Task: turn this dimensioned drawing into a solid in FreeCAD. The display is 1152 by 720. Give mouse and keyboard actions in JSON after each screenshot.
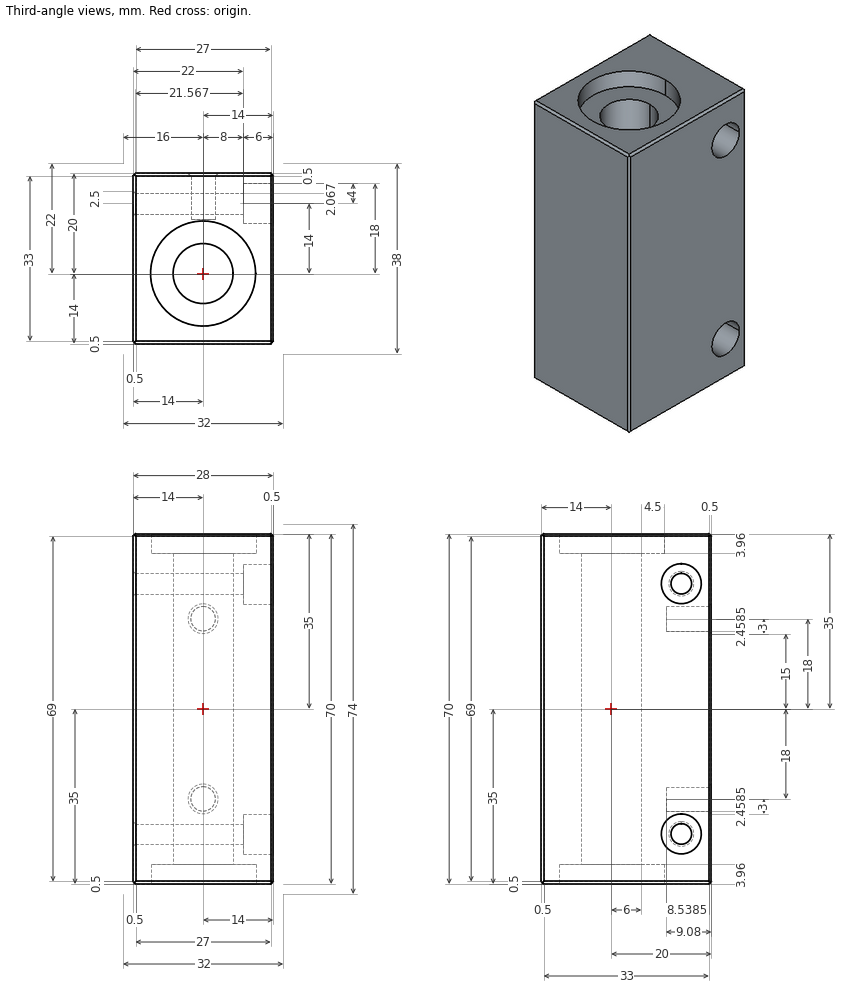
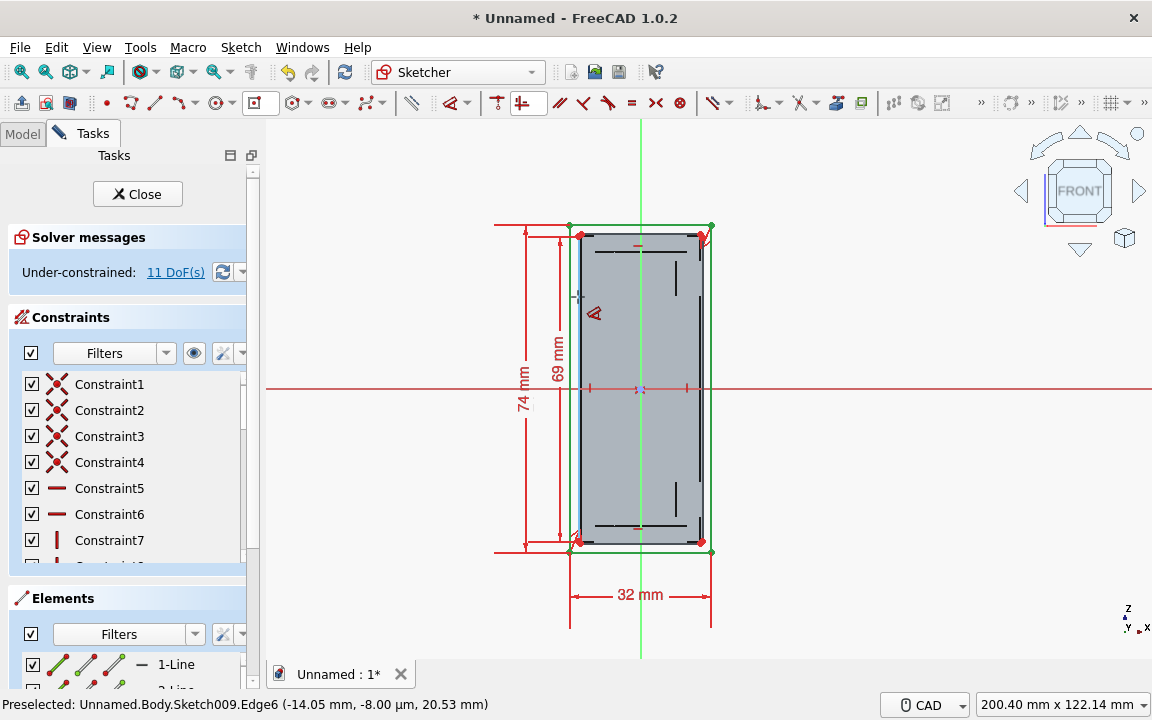
{"action": "scroll", "coordinate": [617, 544], "scroll_direction": "up", "scroll_amount": 3}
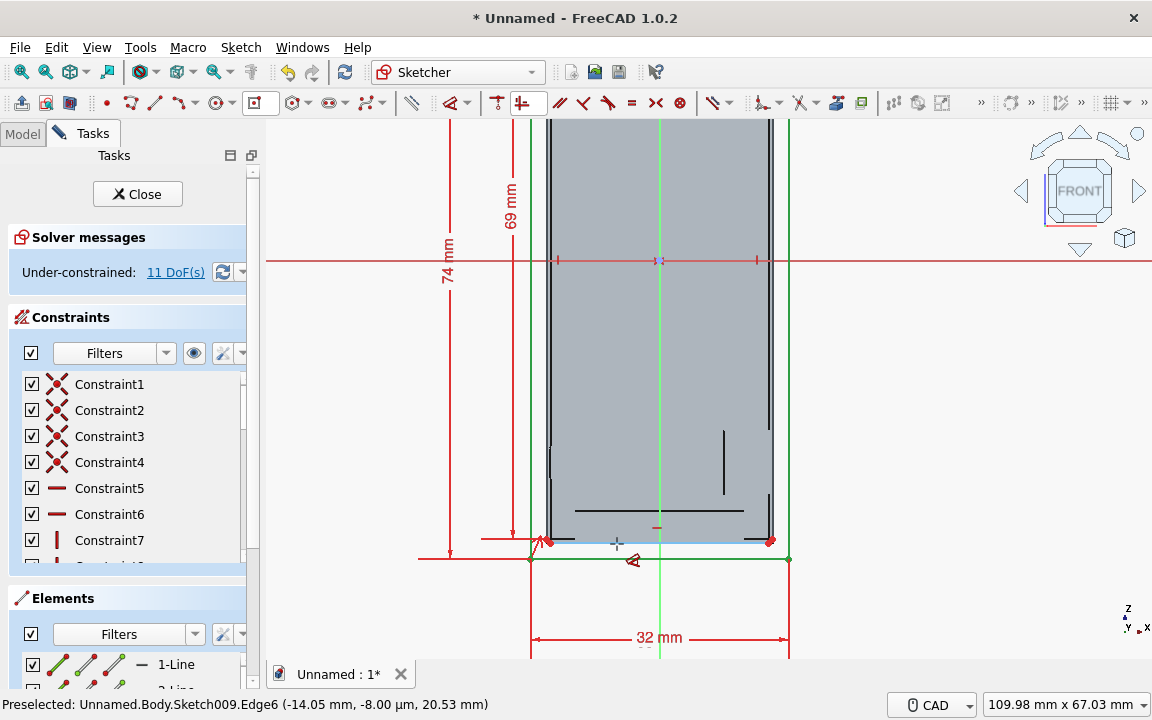
{"action": "left_click", "coordinate": [616, 543]}
{"action": "left_click", "coordinate": [610, 577]}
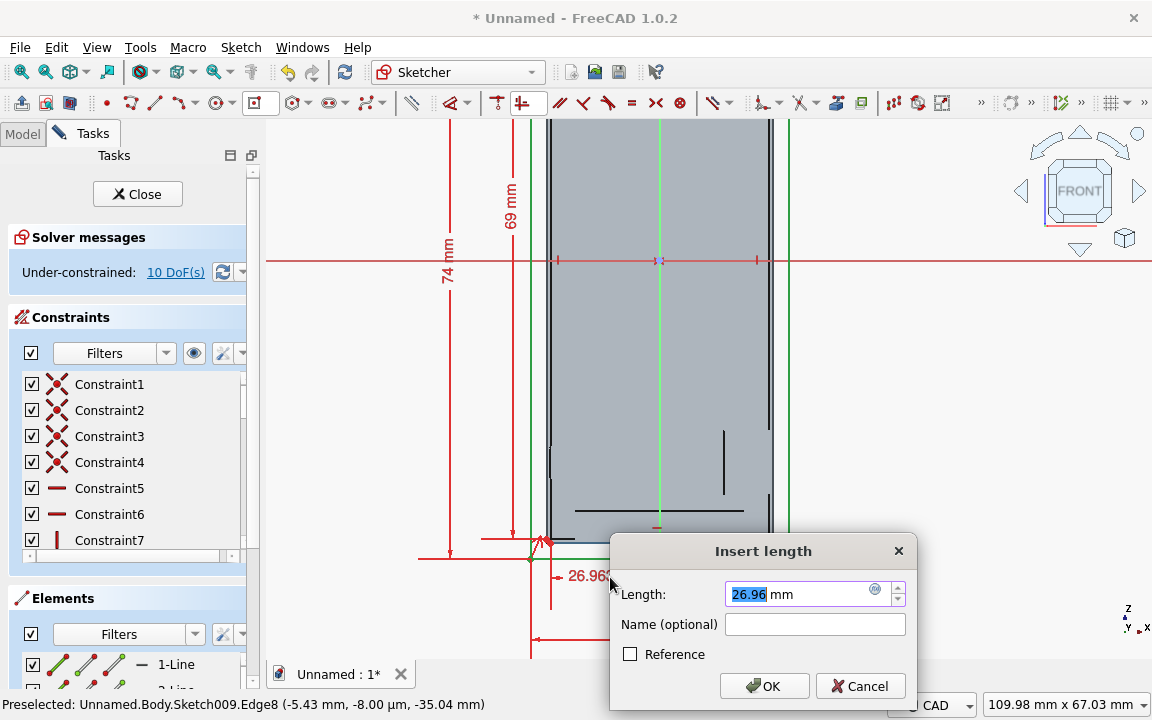
{"action": "type", "text": "27"}
{"action": "key", "text": "Return"}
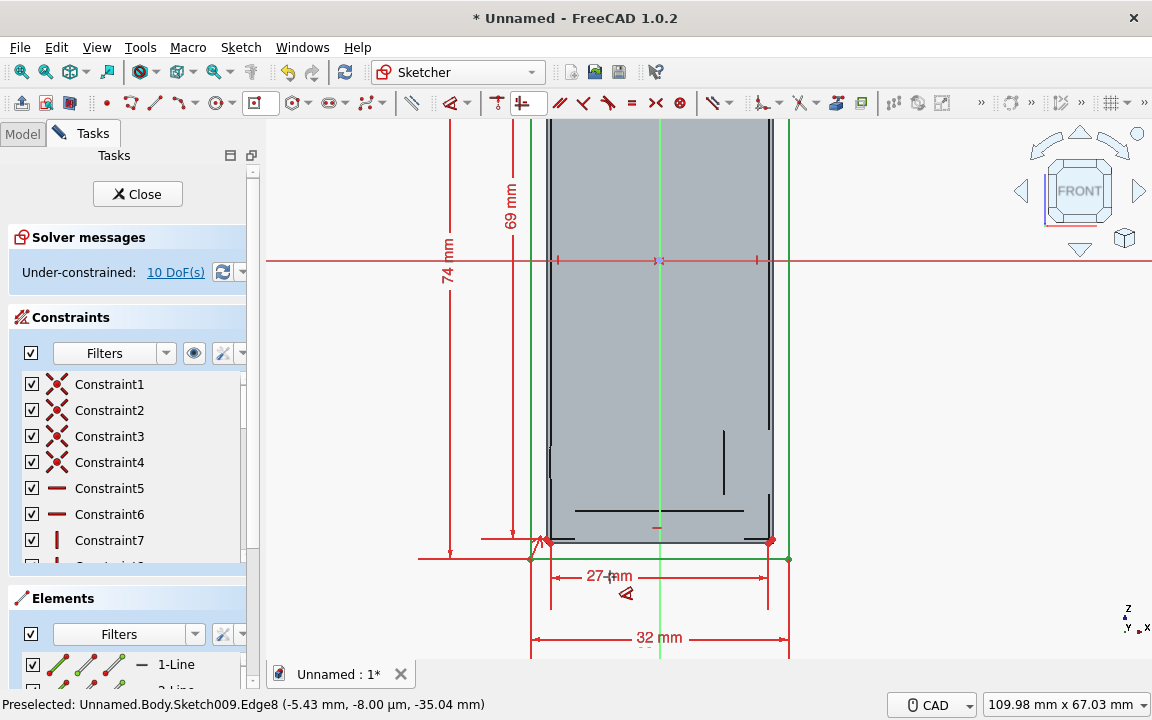
{"action": "left_click", "coordinate": [773, 373]}
{"action": "left_click", "coordinate": [807, 343]}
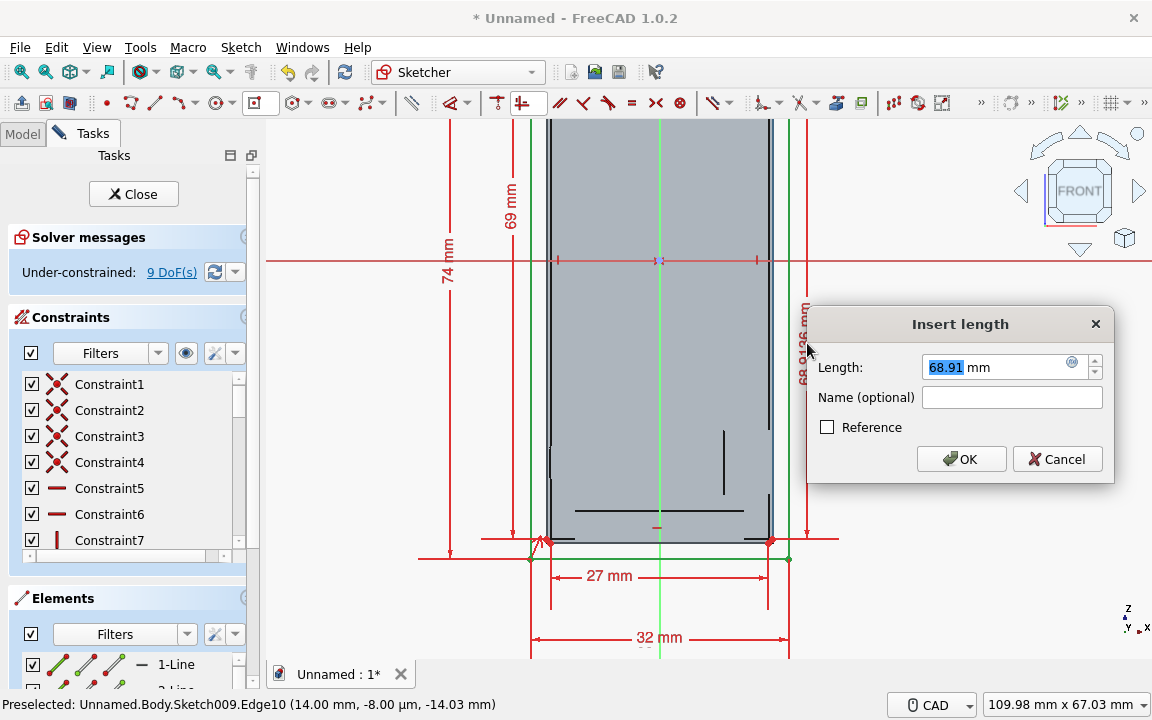
{"action": "type", "text": "69"}
{"action": "key", "text": "Return"}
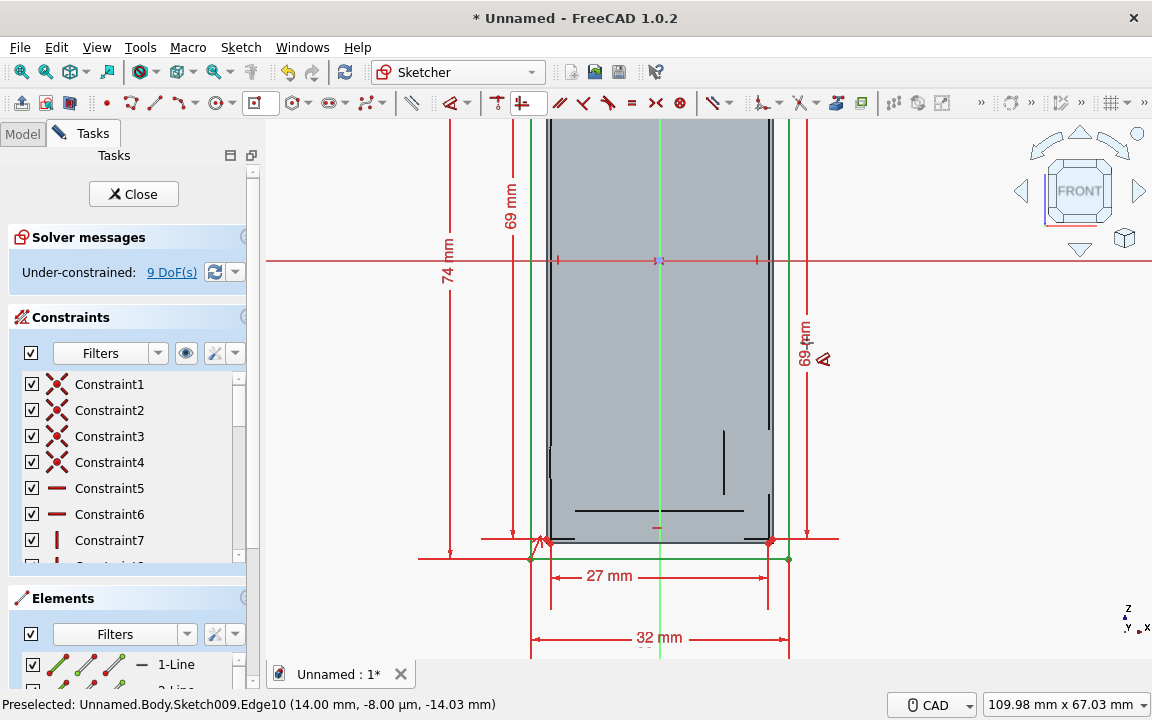
{"action": "scroll", "coordinate": [617, 545], "scroll_direction": "down", "scroll_amount": 3}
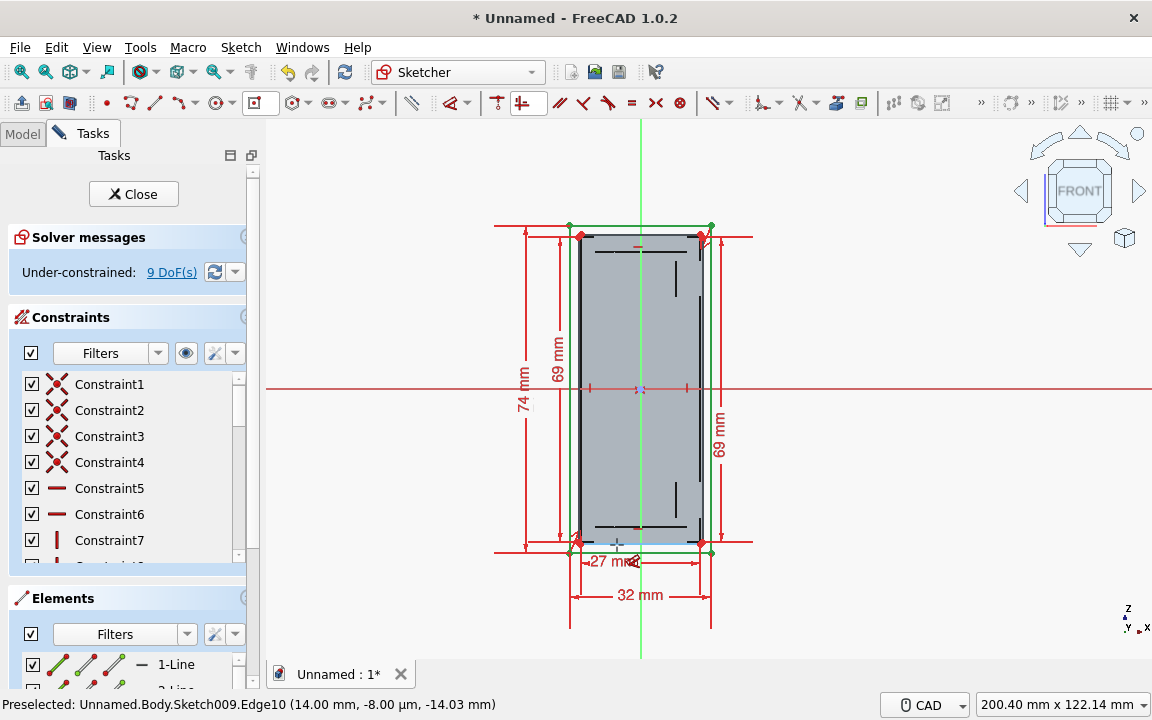
{"action": "scroll", "coordinate": [665, 235], "scroll_direction": "up", "scroll_amount": 3}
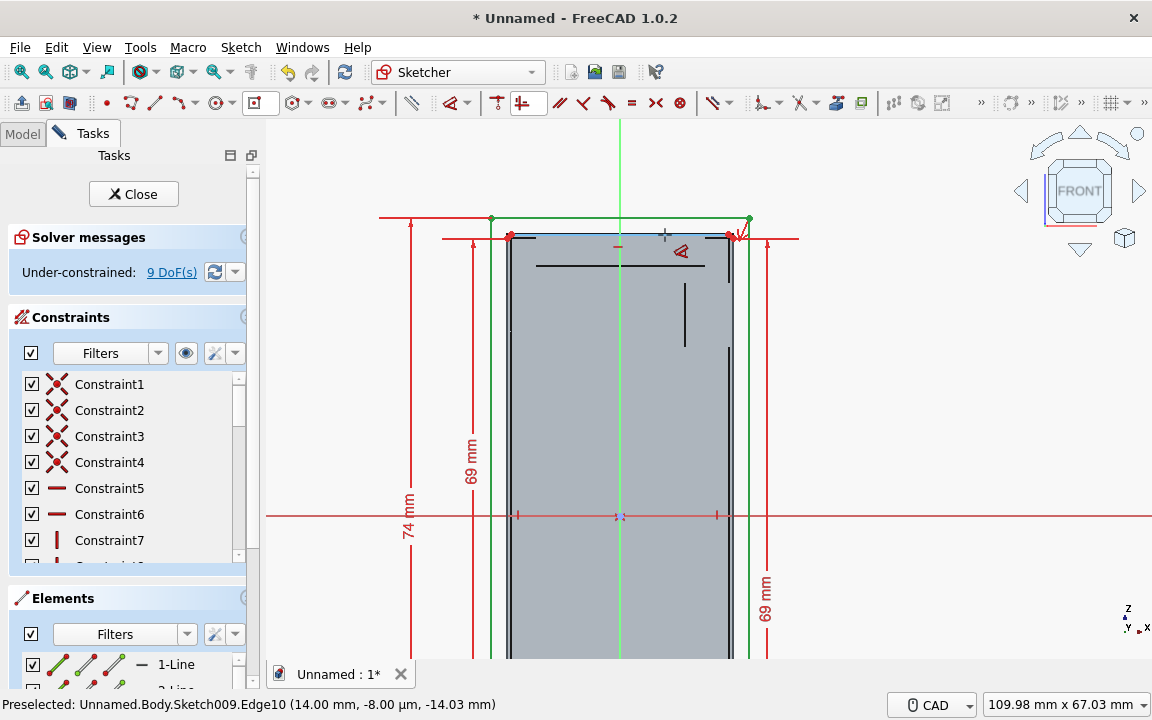
{"action": "left_click", "coordinate": [664, 235]}
{"action": "left_click", "coordinate": [570, 201]}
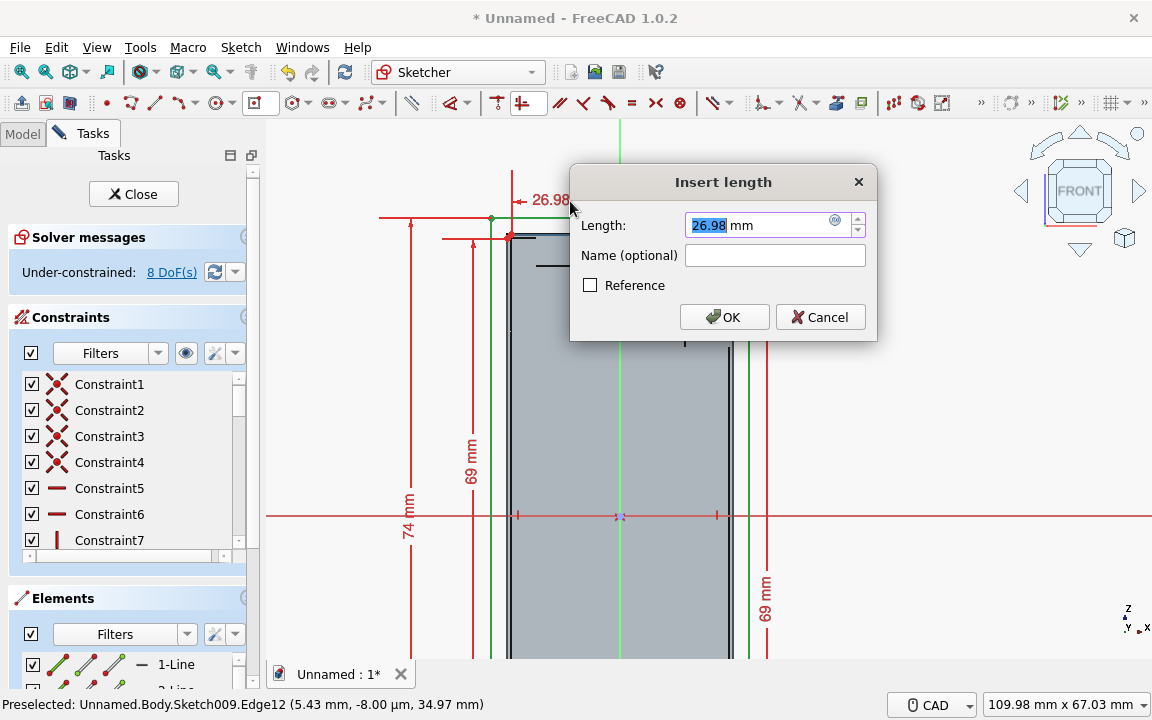
{"action": "type", "text": "27"}
{"action": "key", "text": "Return"}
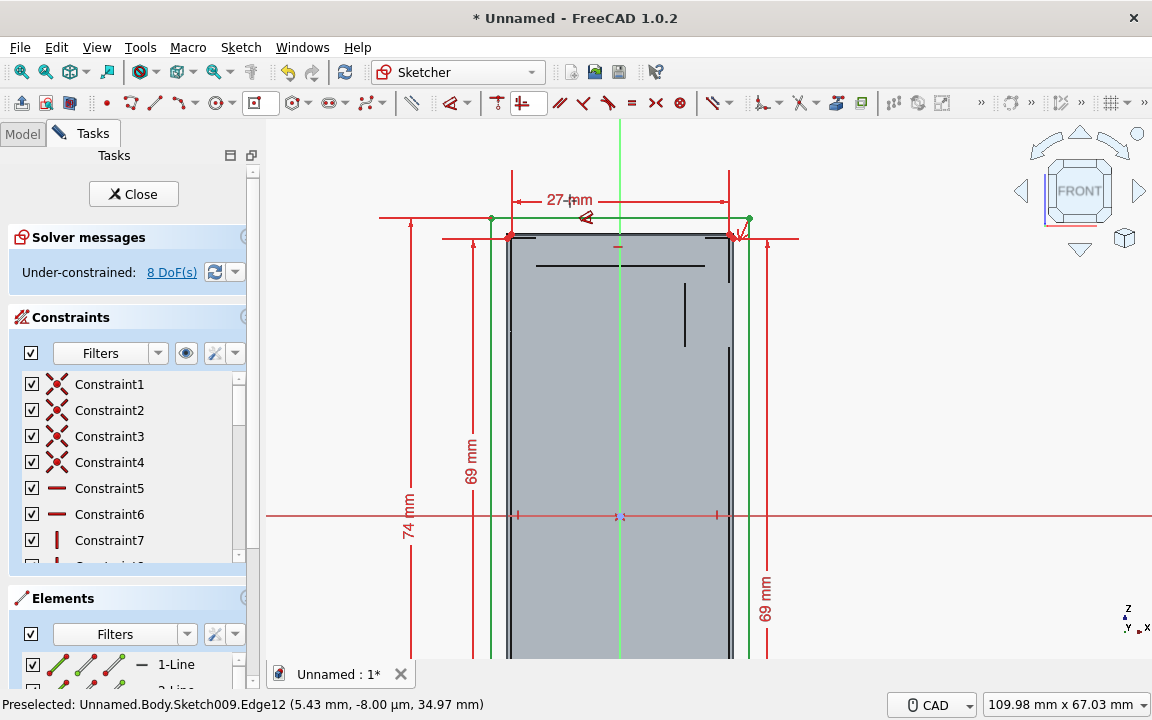
{"action": "scroll", "coordinate": [507, 239], "scroll_direction": "up", "scroll_amount": 4}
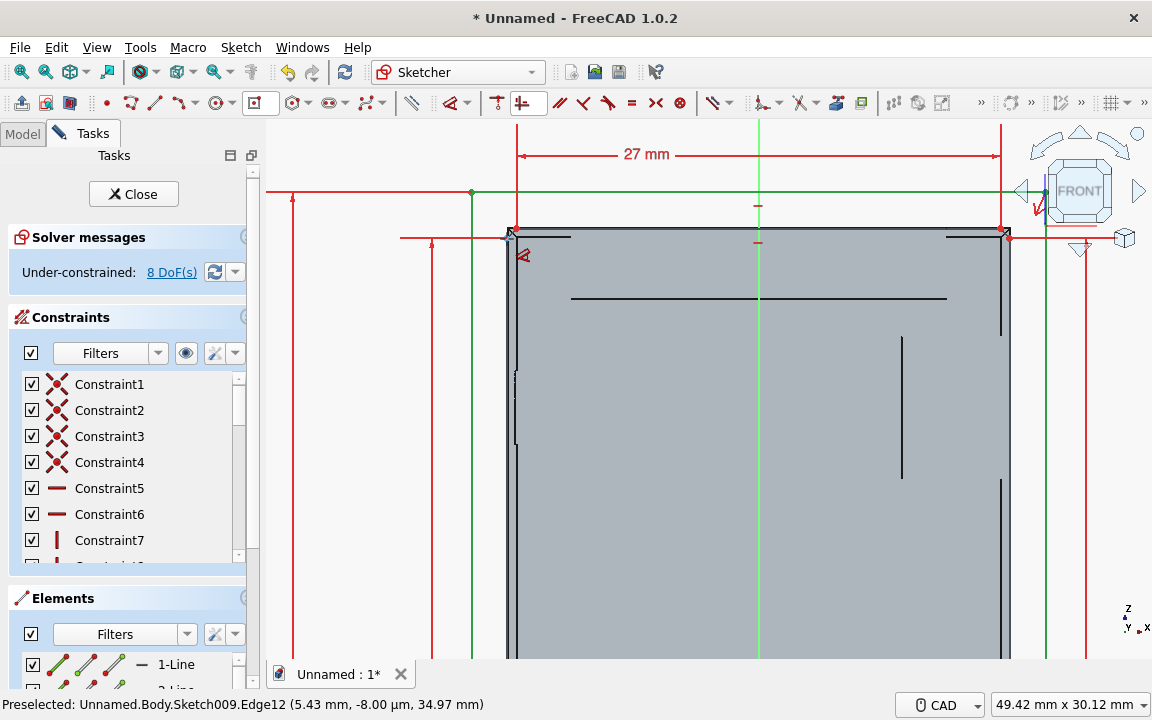
{"action": "left_click", "coordinate": [507, 238]}
{"action": "left_click", "coordinate": [575, 156]}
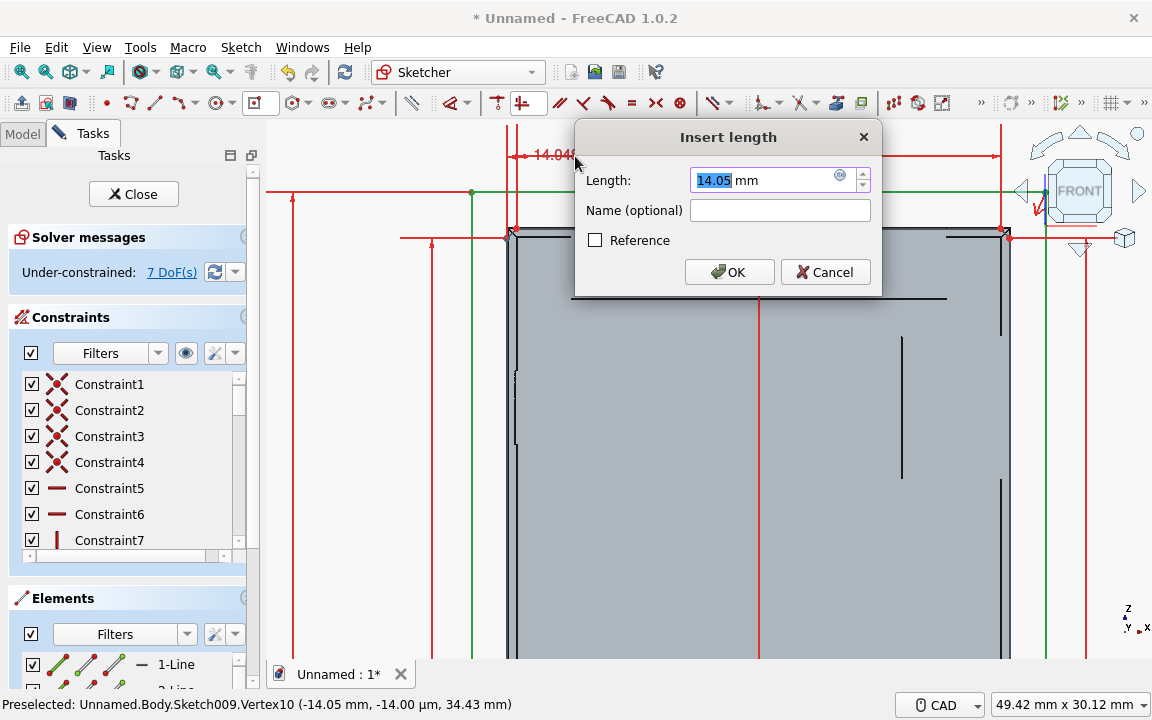
{"action": "type", "text": "14"}
{"action": "key", "text": "Return"}